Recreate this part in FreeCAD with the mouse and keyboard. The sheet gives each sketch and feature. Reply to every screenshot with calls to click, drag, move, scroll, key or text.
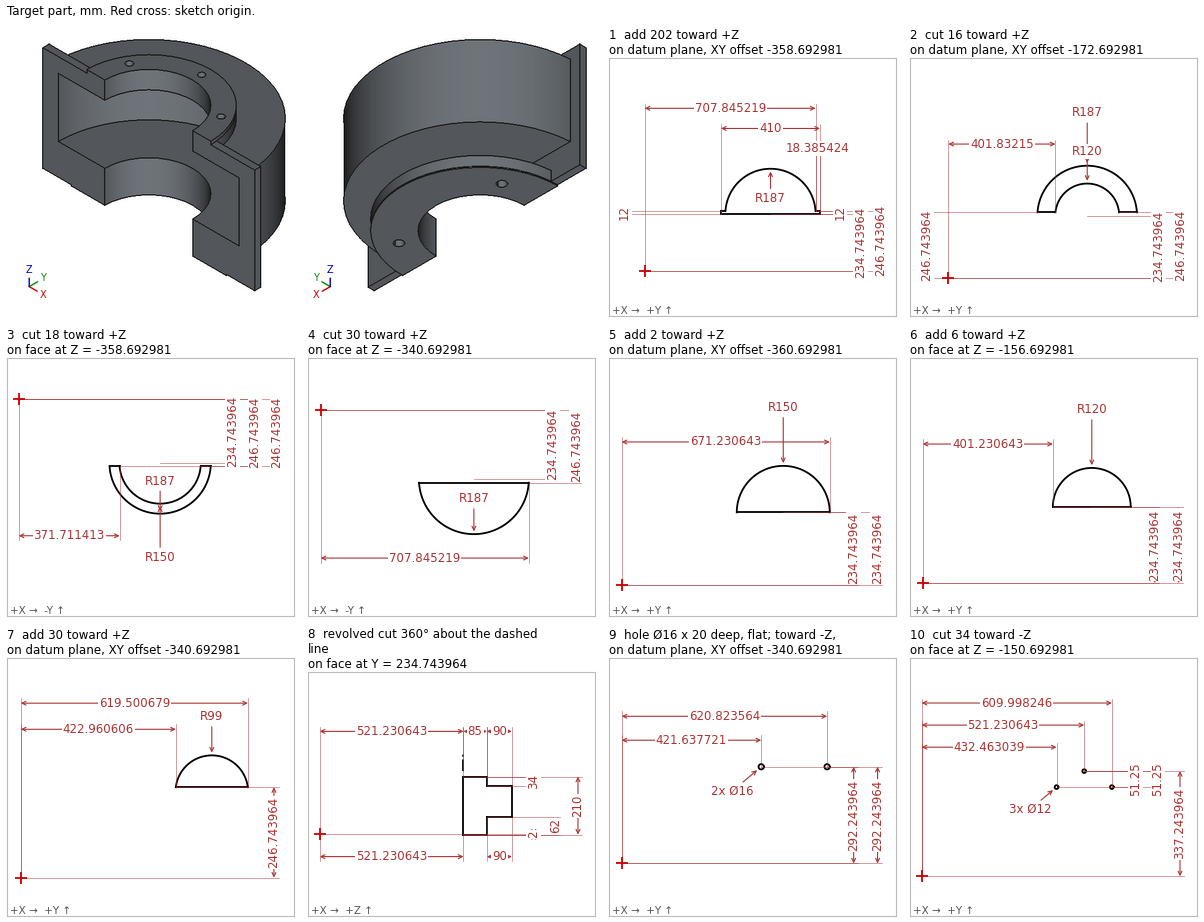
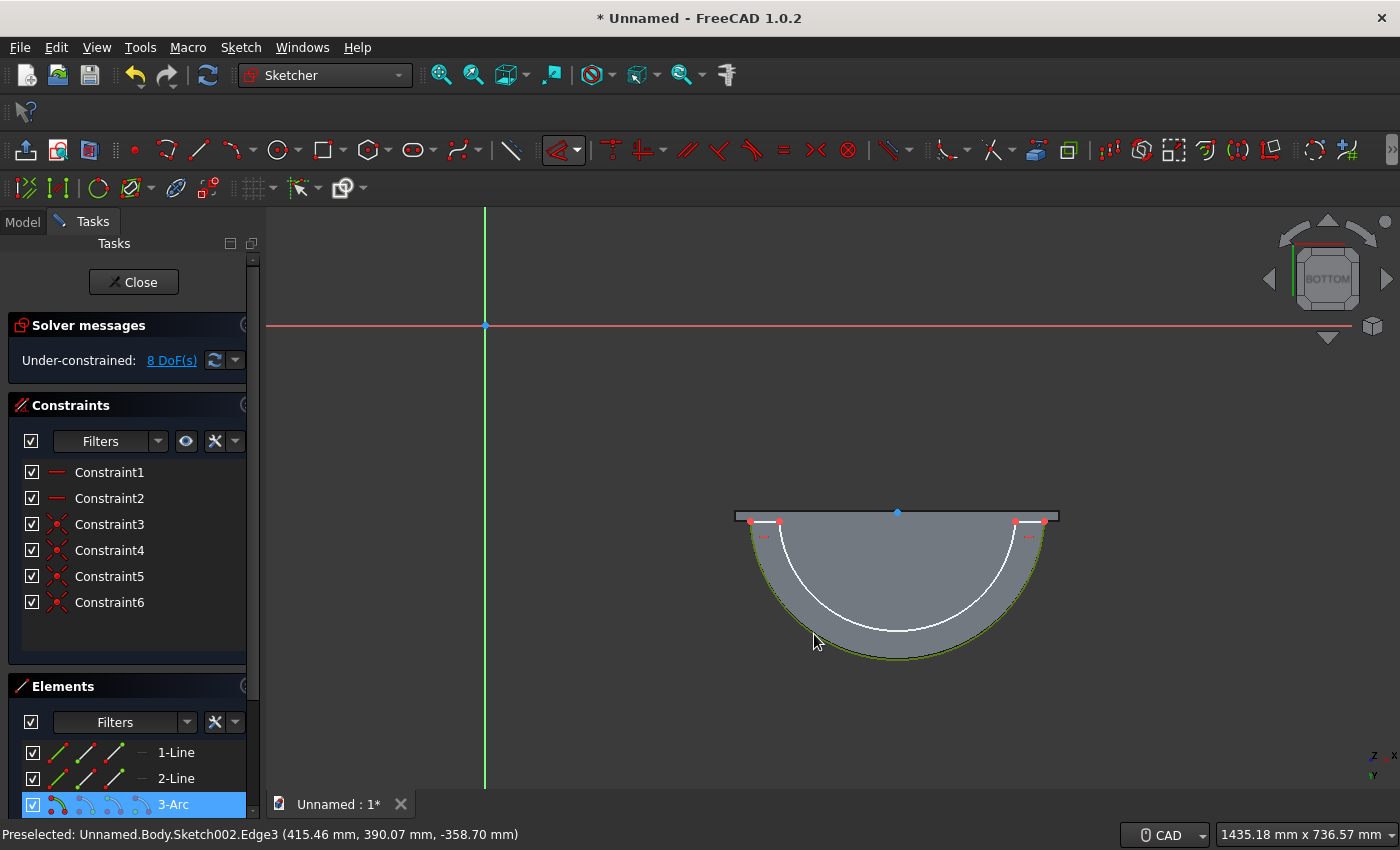
click(831, 611)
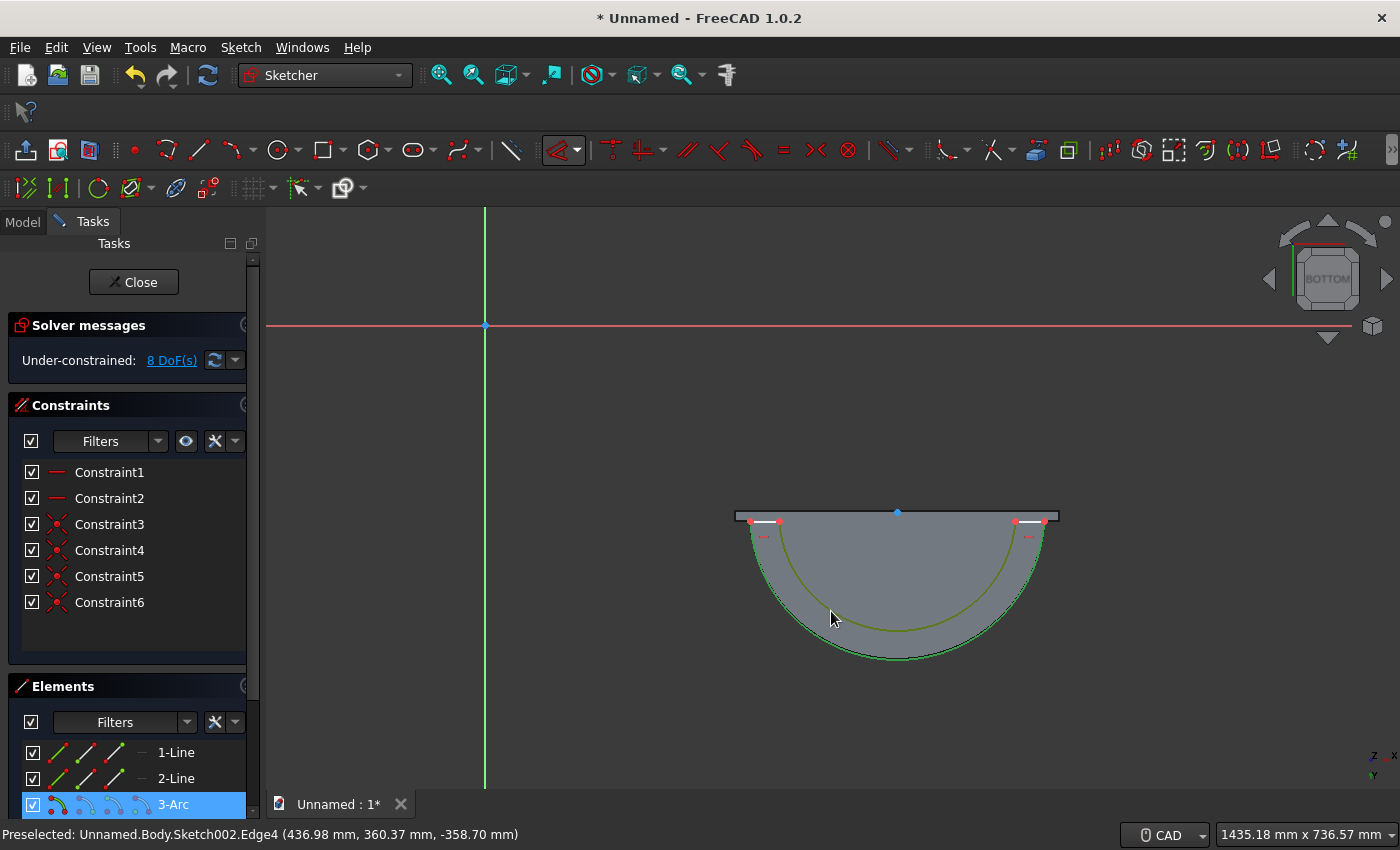
key(c)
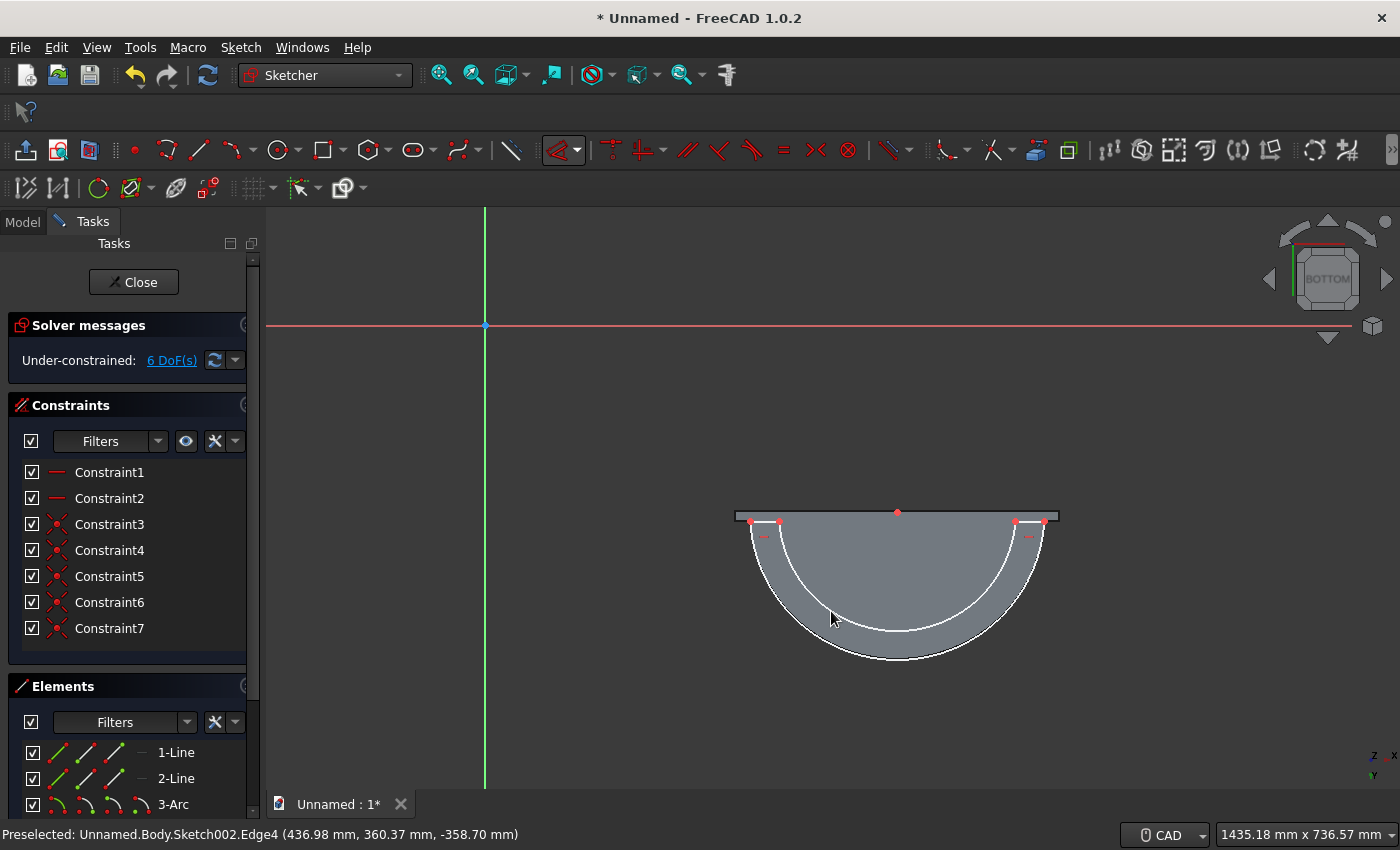
key(d)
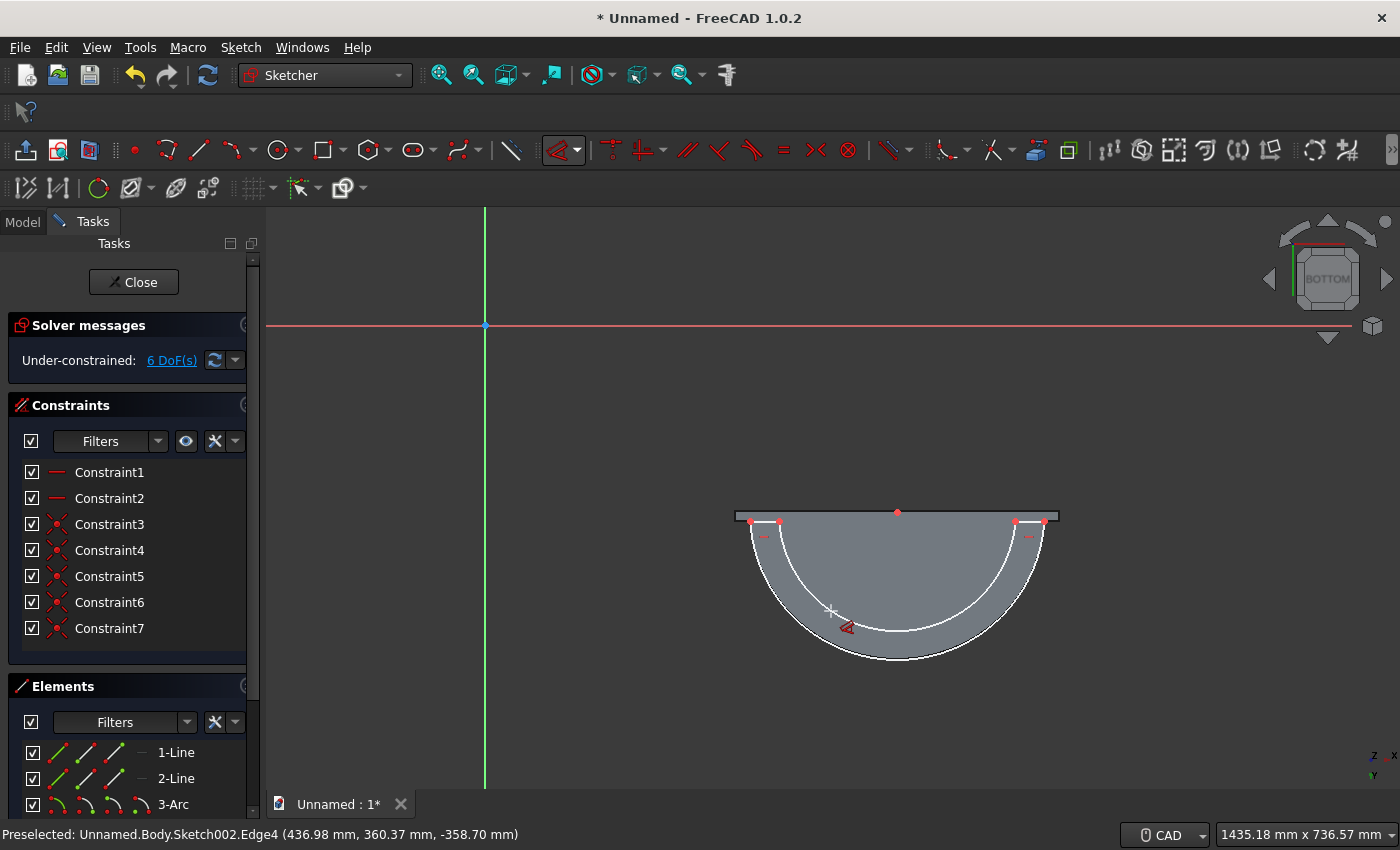
click(814, 634)
click(796, 660)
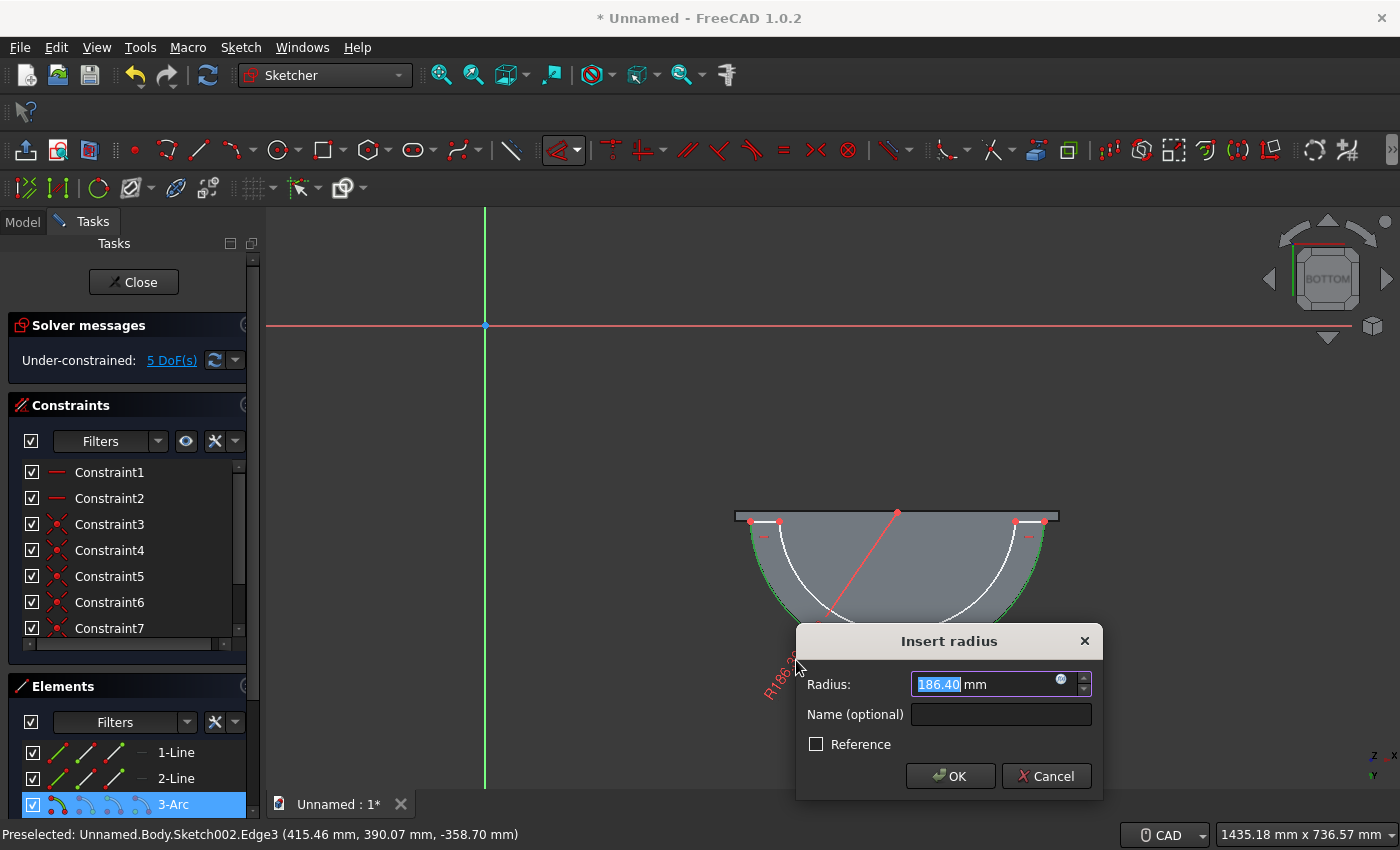
text(187)
key(Return)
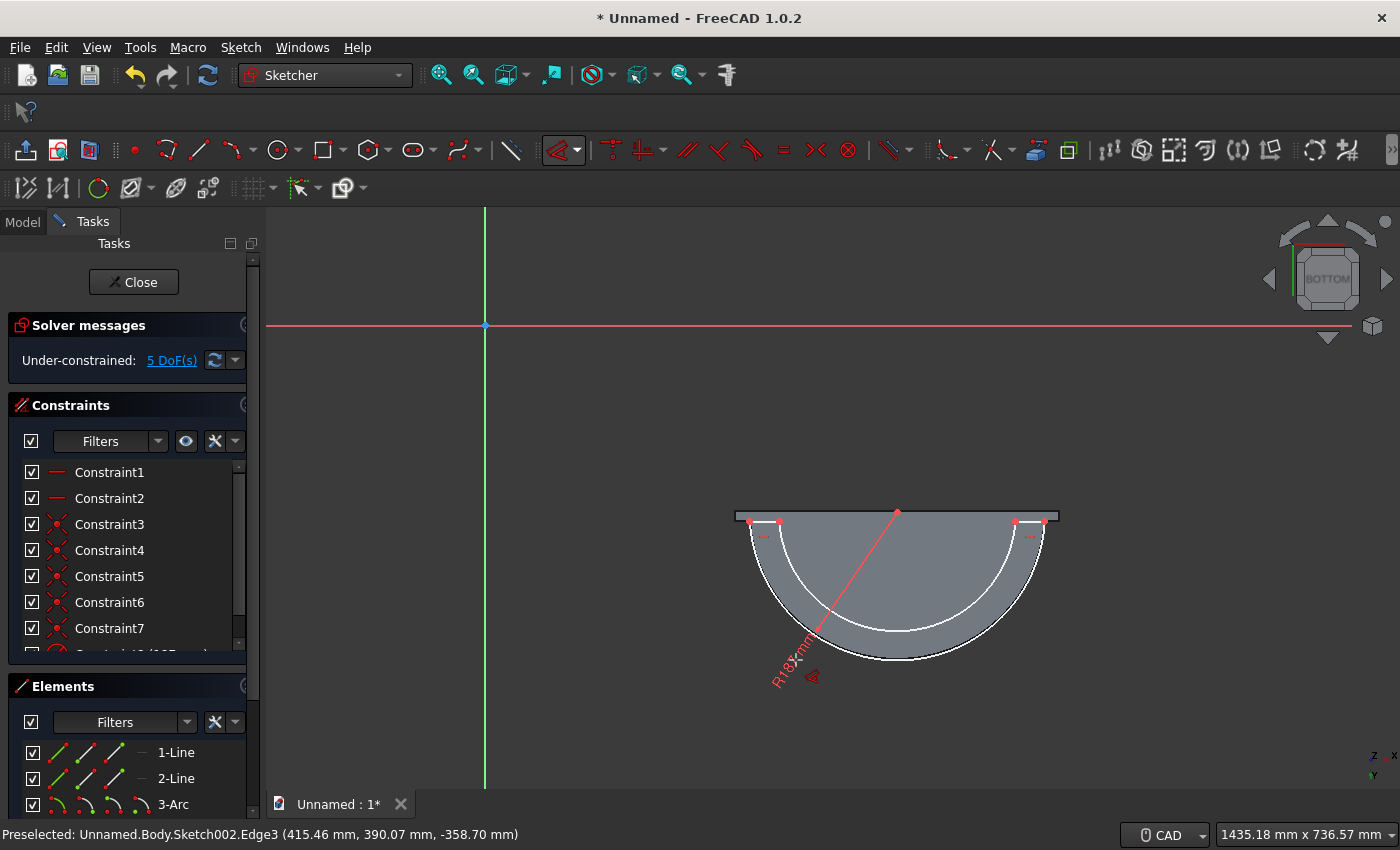
click(831, 611)
click(747, 509)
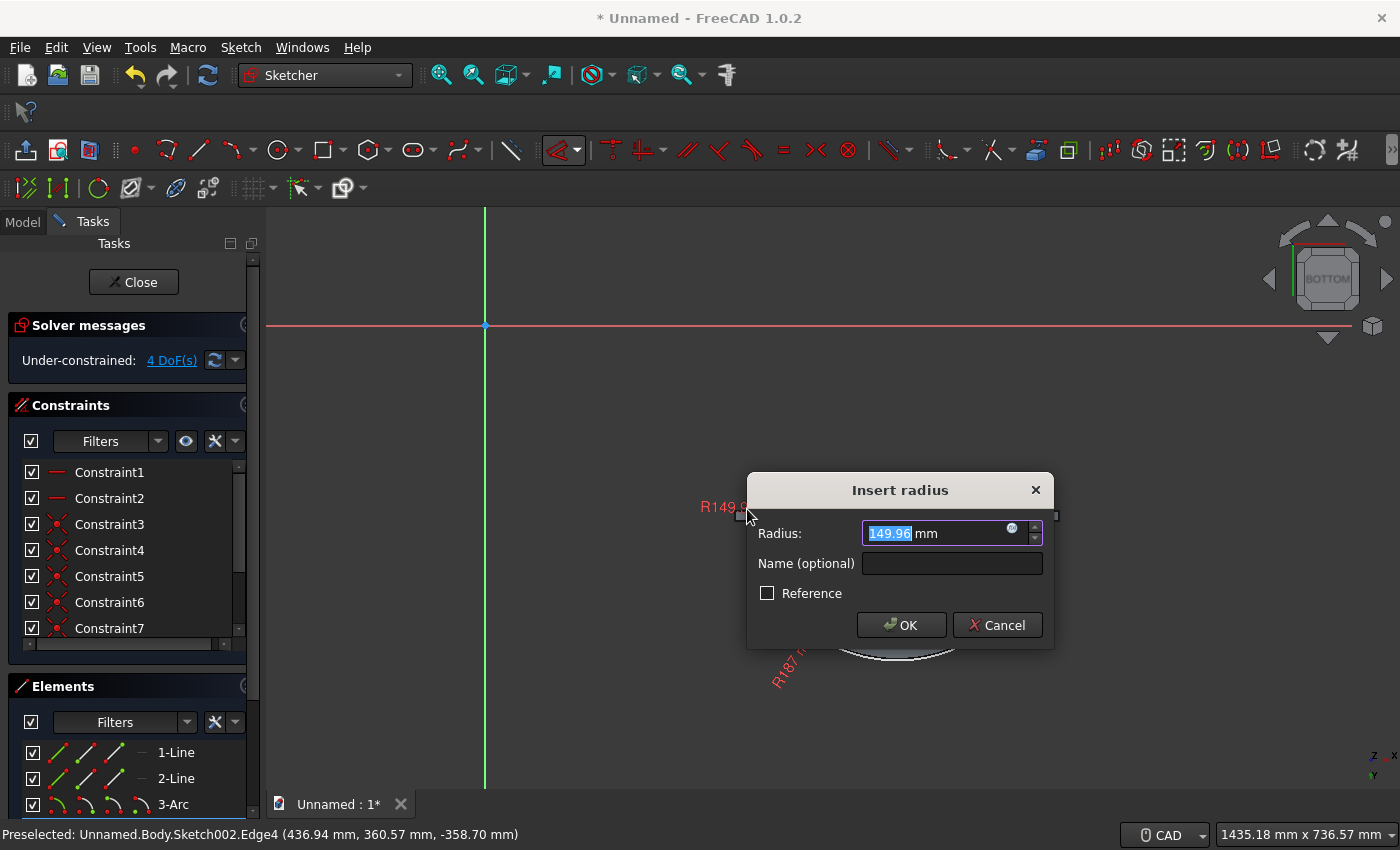
text(150)
key(Return)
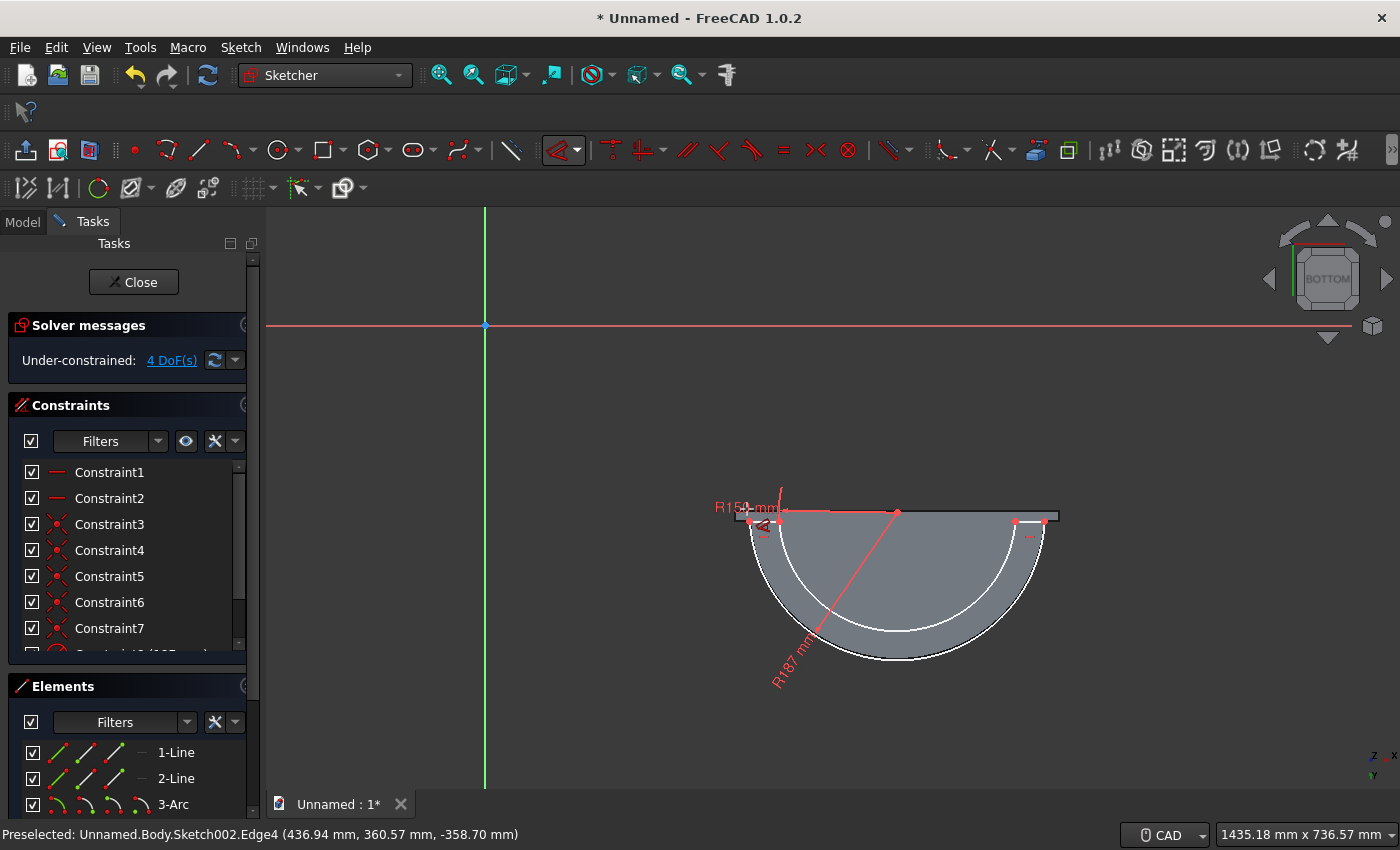
click(779, 522)
click(632, 292)